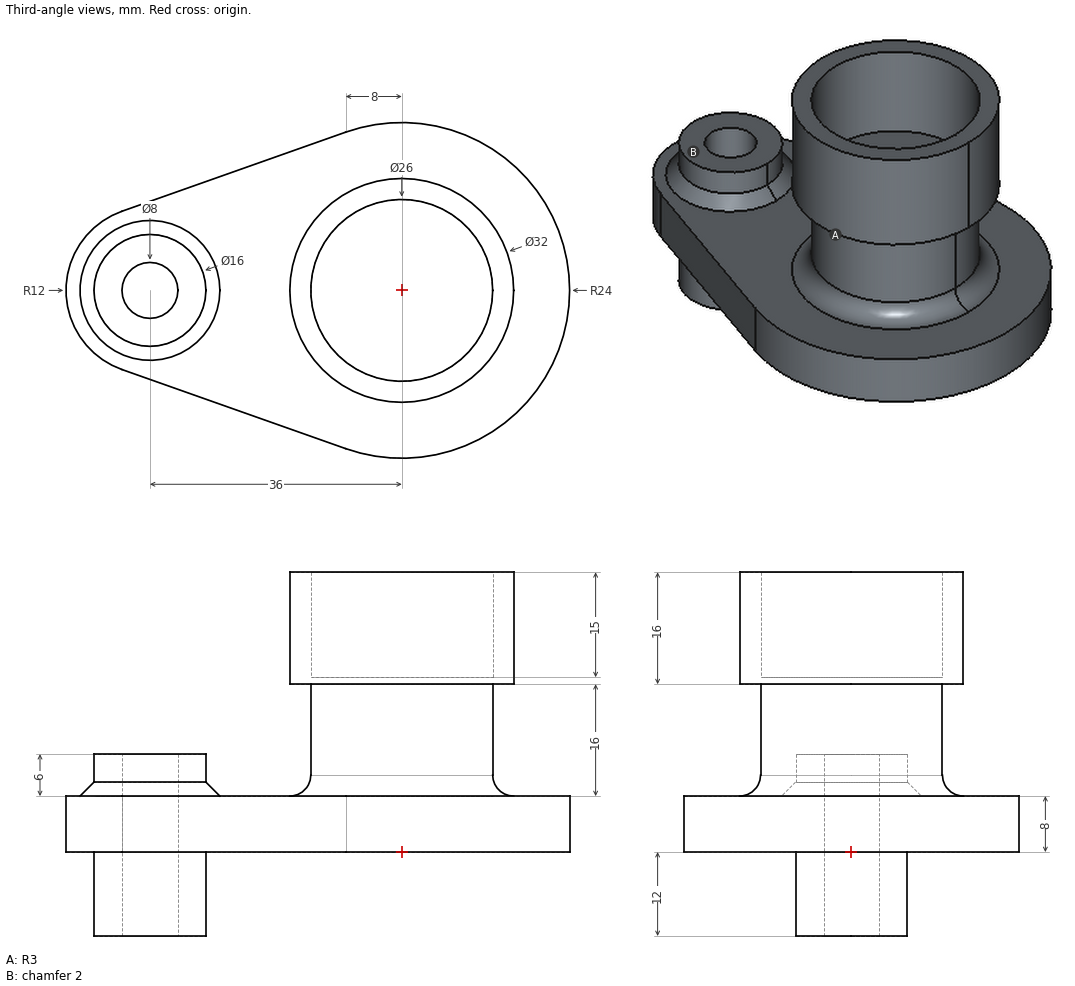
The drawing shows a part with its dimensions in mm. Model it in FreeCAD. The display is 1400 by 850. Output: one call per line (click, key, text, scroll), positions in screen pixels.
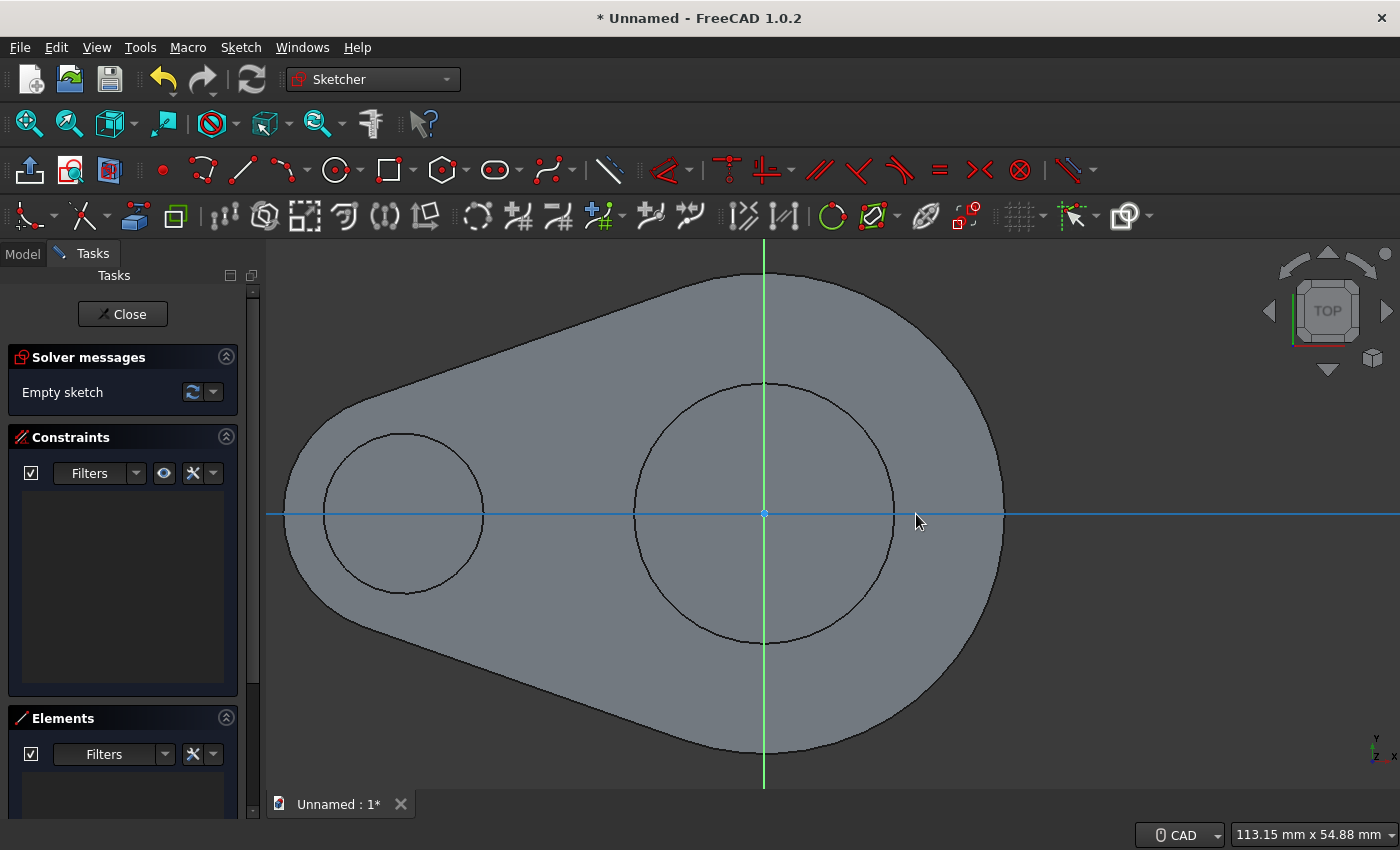
click(336, 170)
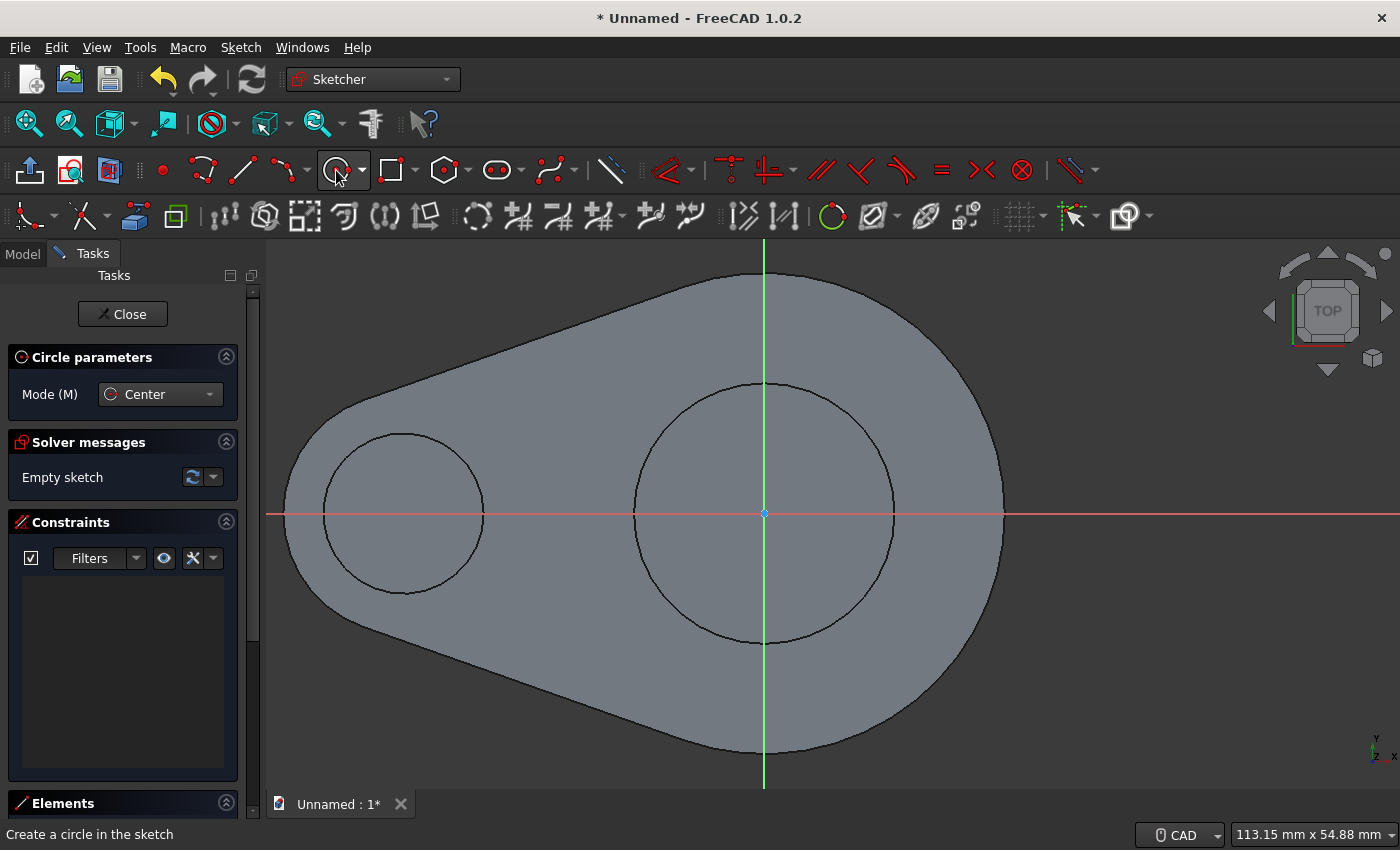
click(764, 514)
move(878, 400)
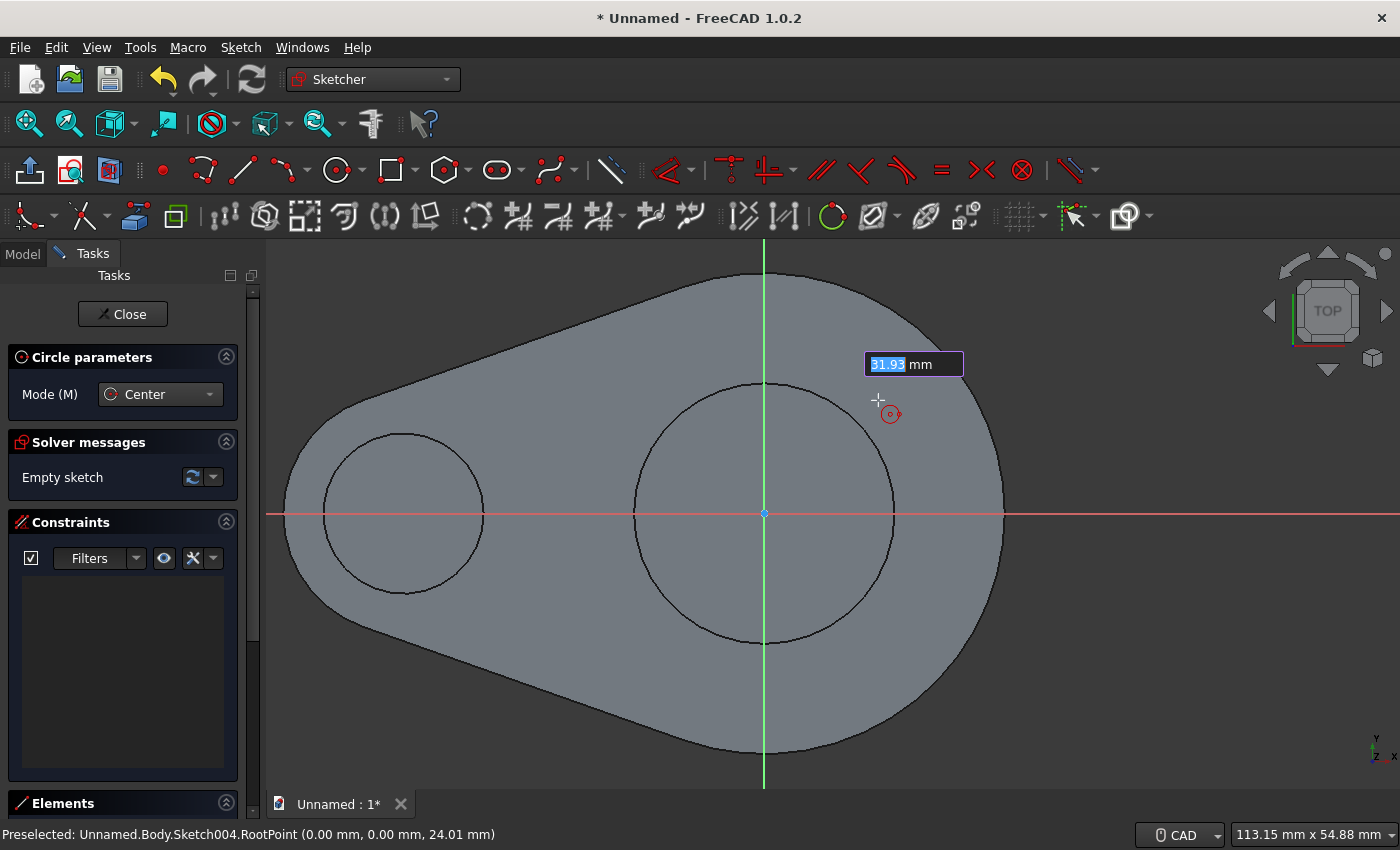
text(32)
key(Return)
key(Escape)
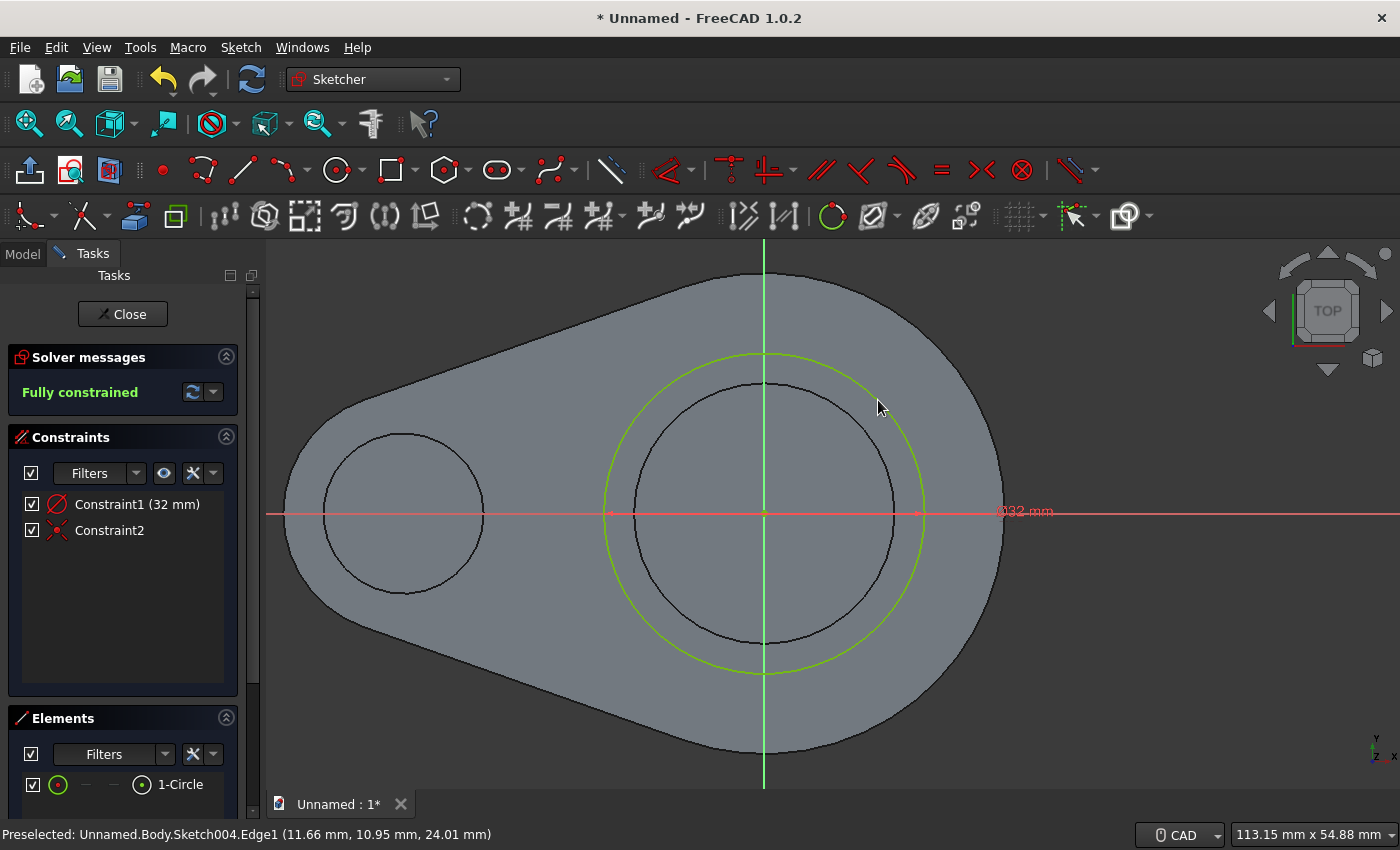
click(123, 314)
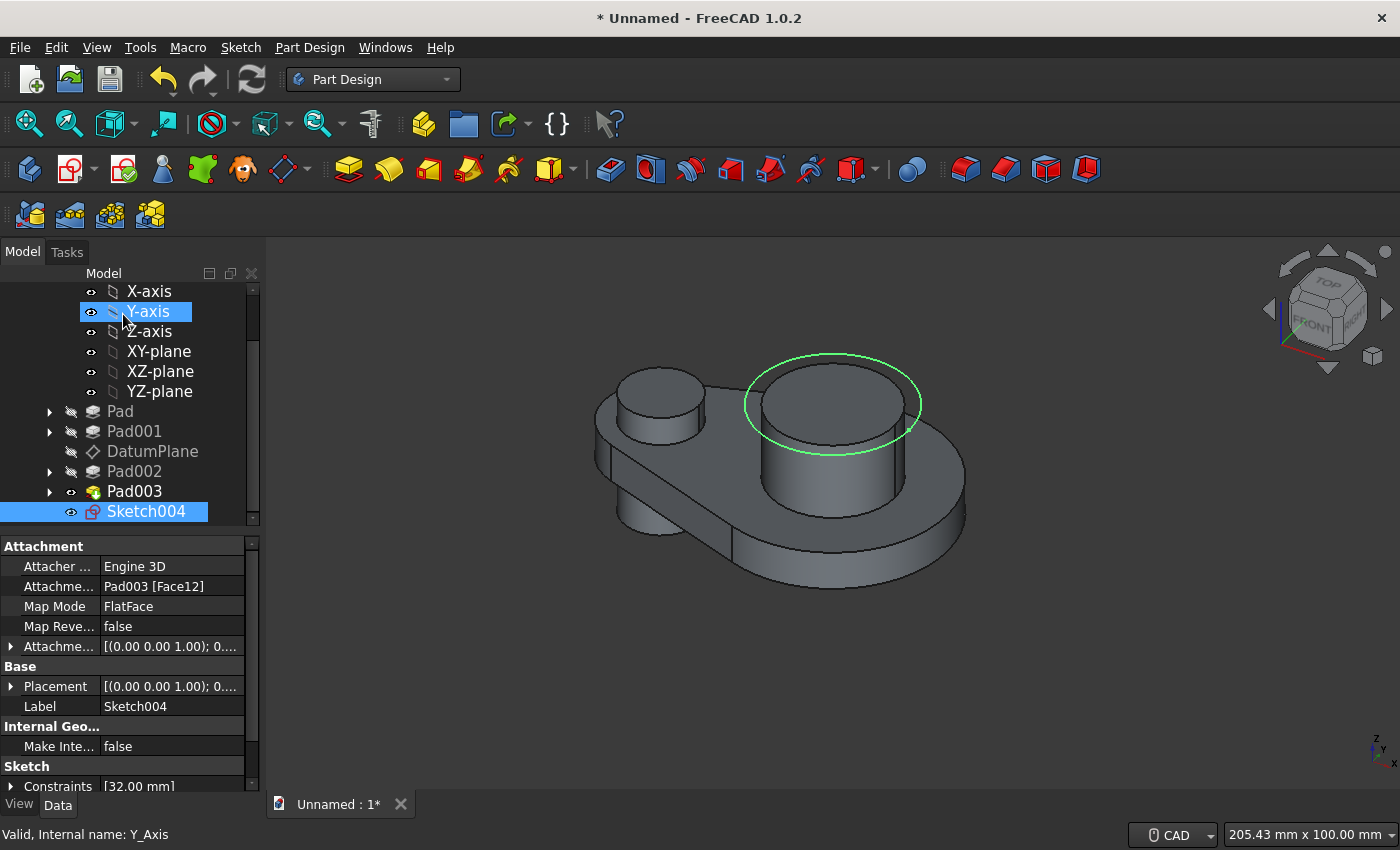
click(350, 170)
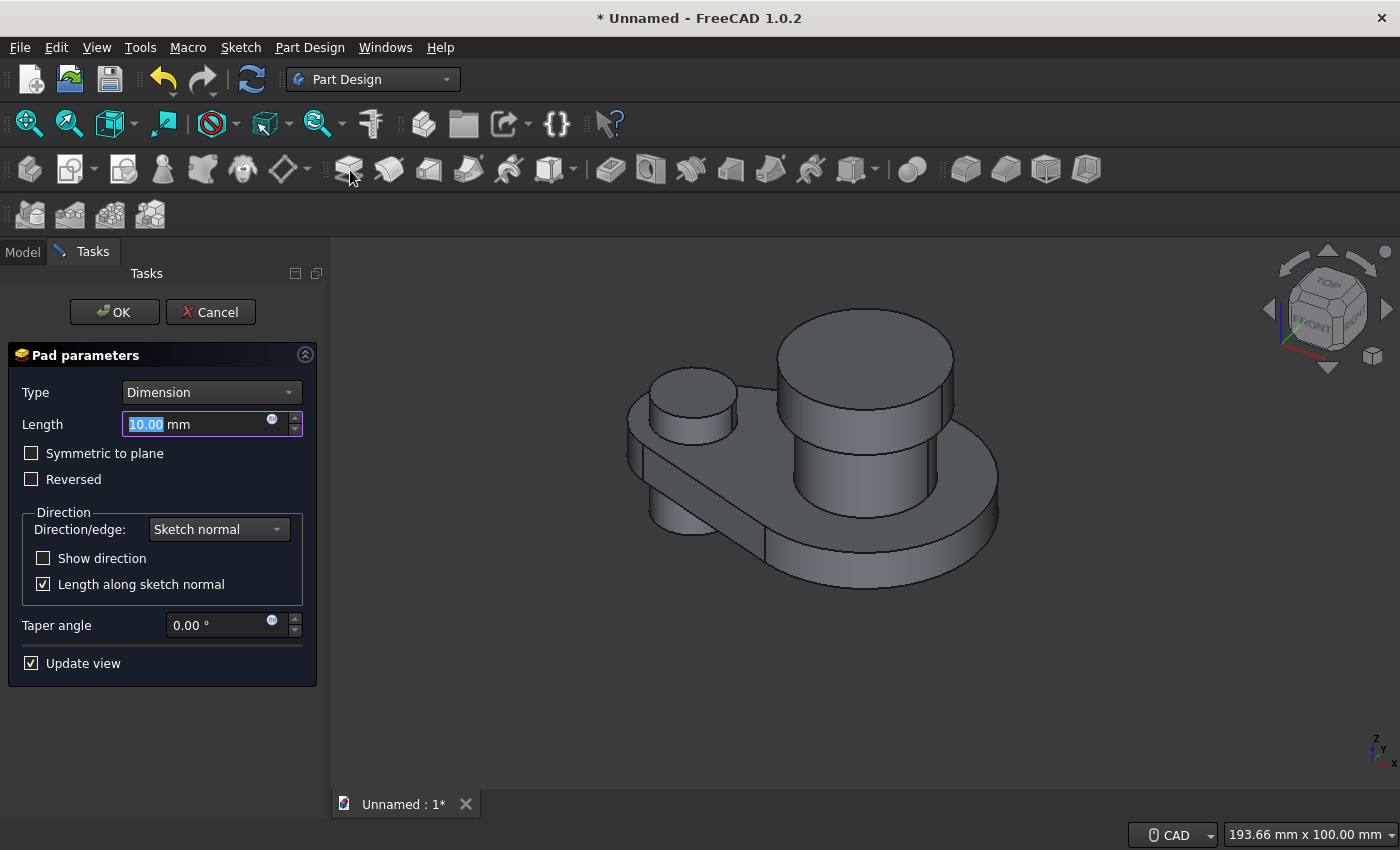
text(16)
key(Tab)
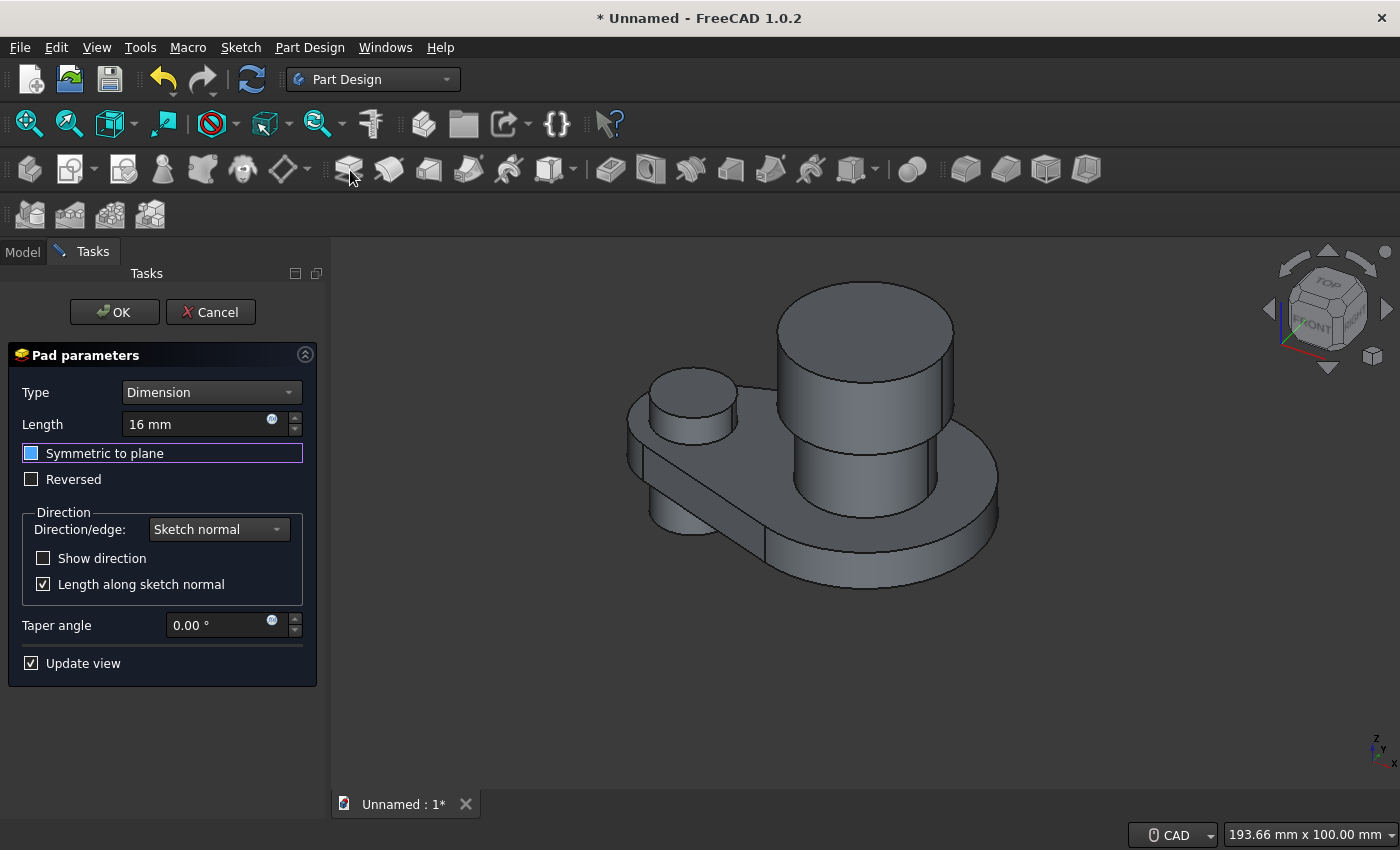
click(115, 312)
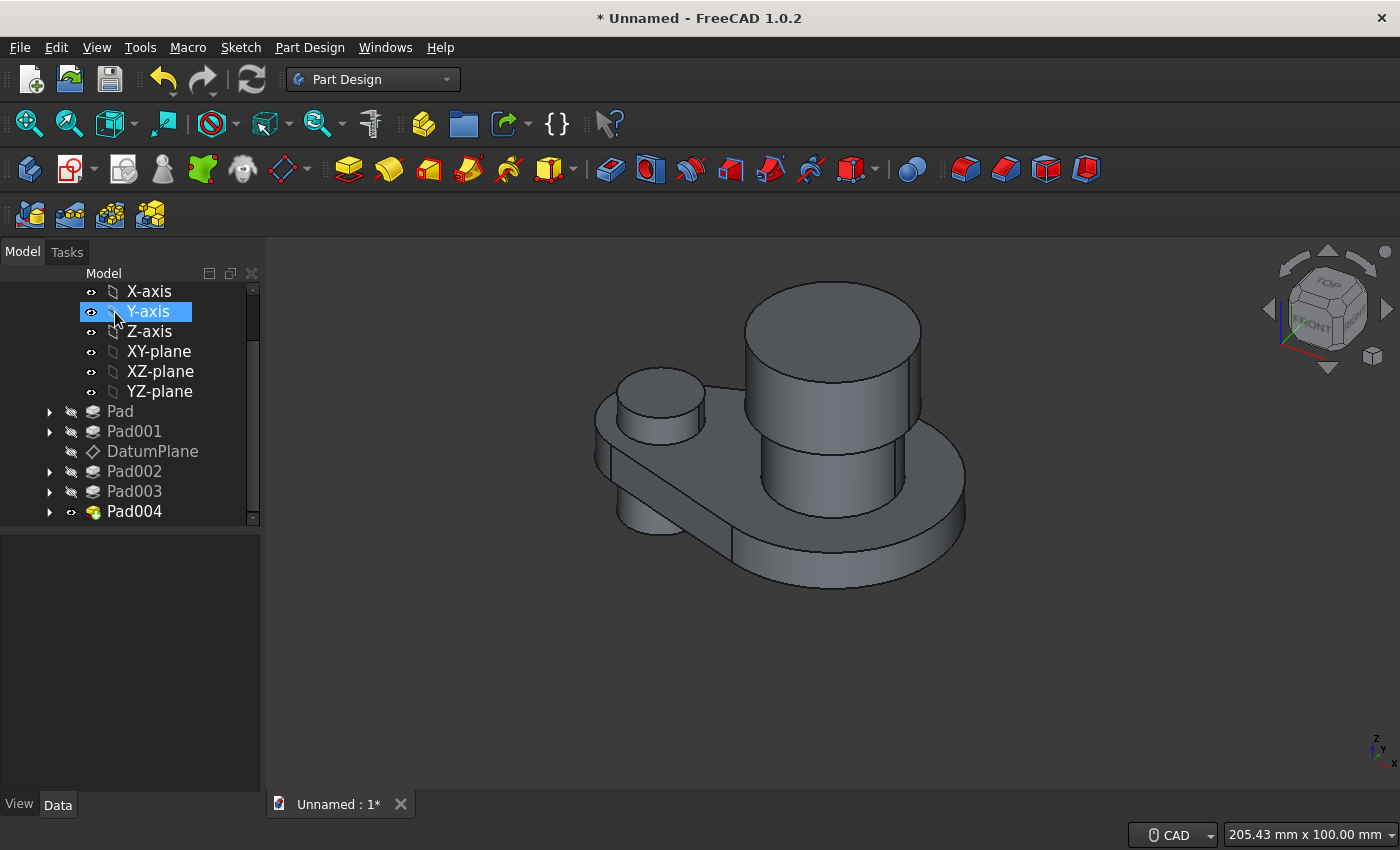
click(30, 124)